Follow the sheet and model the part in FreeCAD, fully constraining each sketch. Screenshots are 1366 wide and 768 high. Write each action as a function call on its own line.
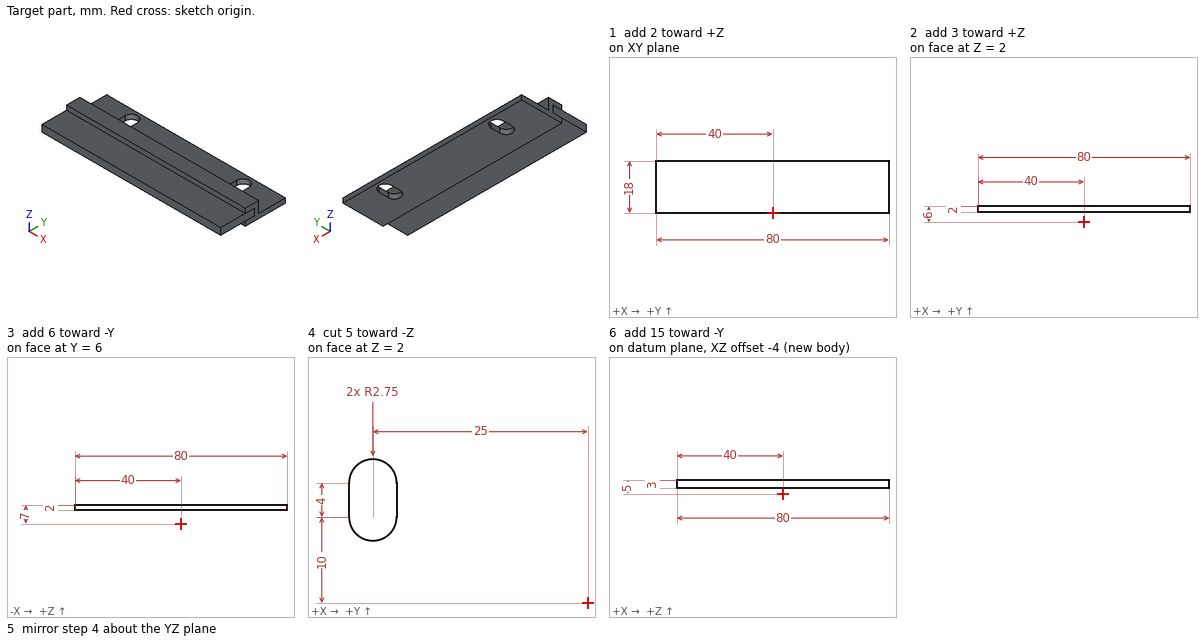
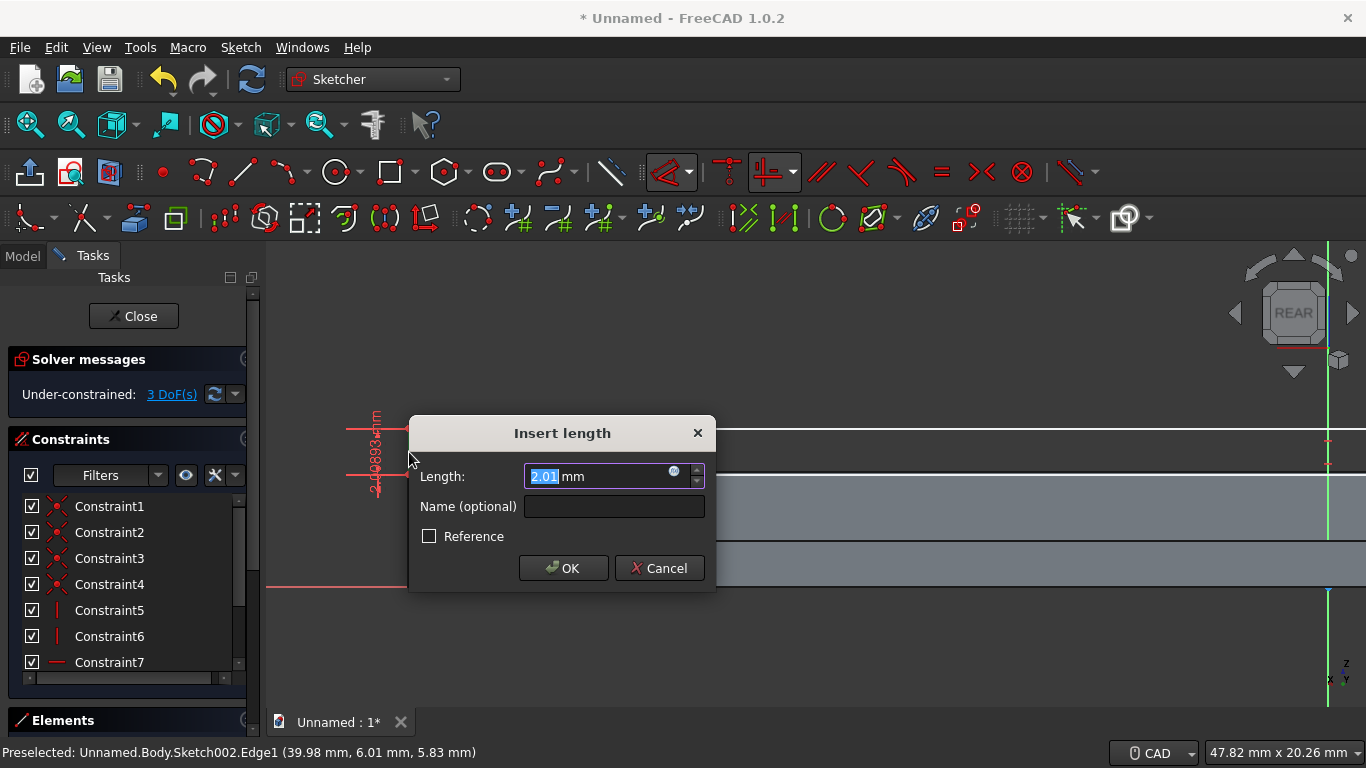
text(2)
key(Return)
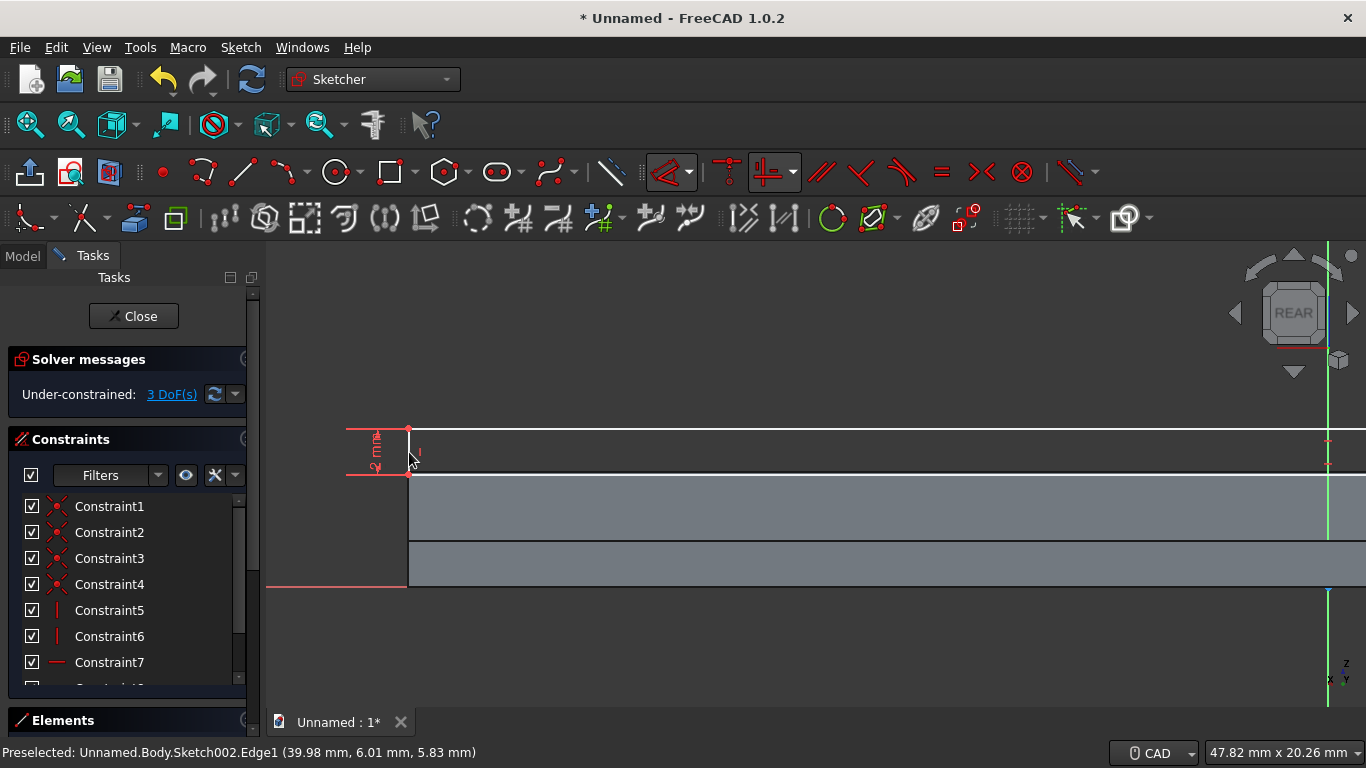
click(961, 475)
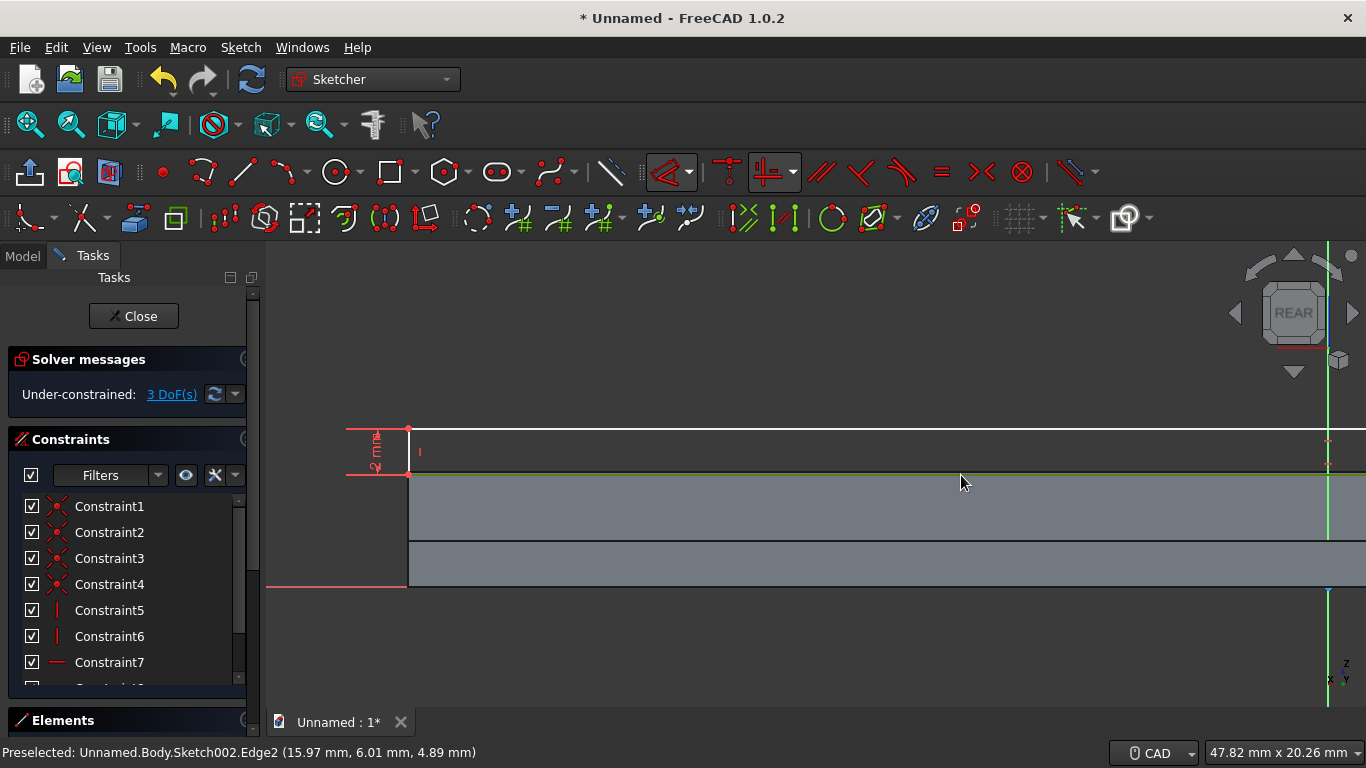
key(l)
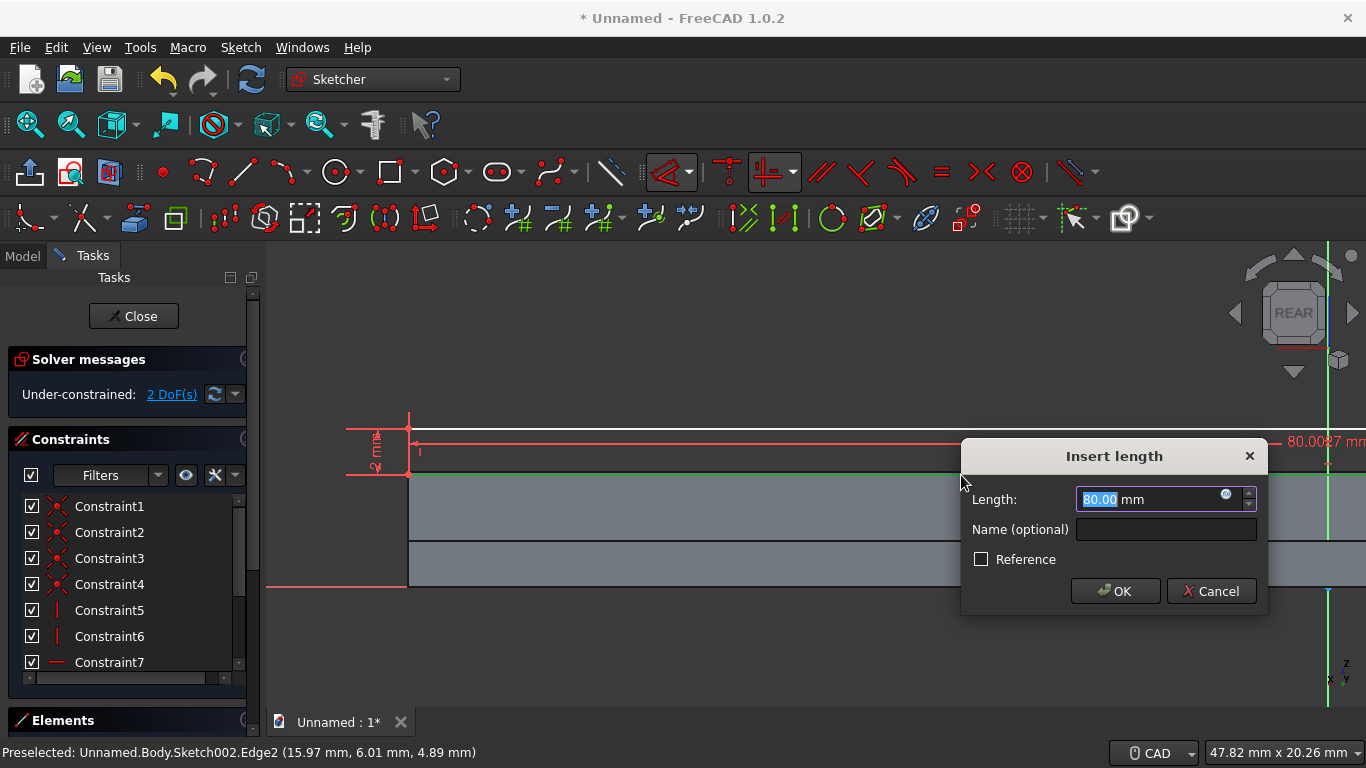
text(80)
key(Return)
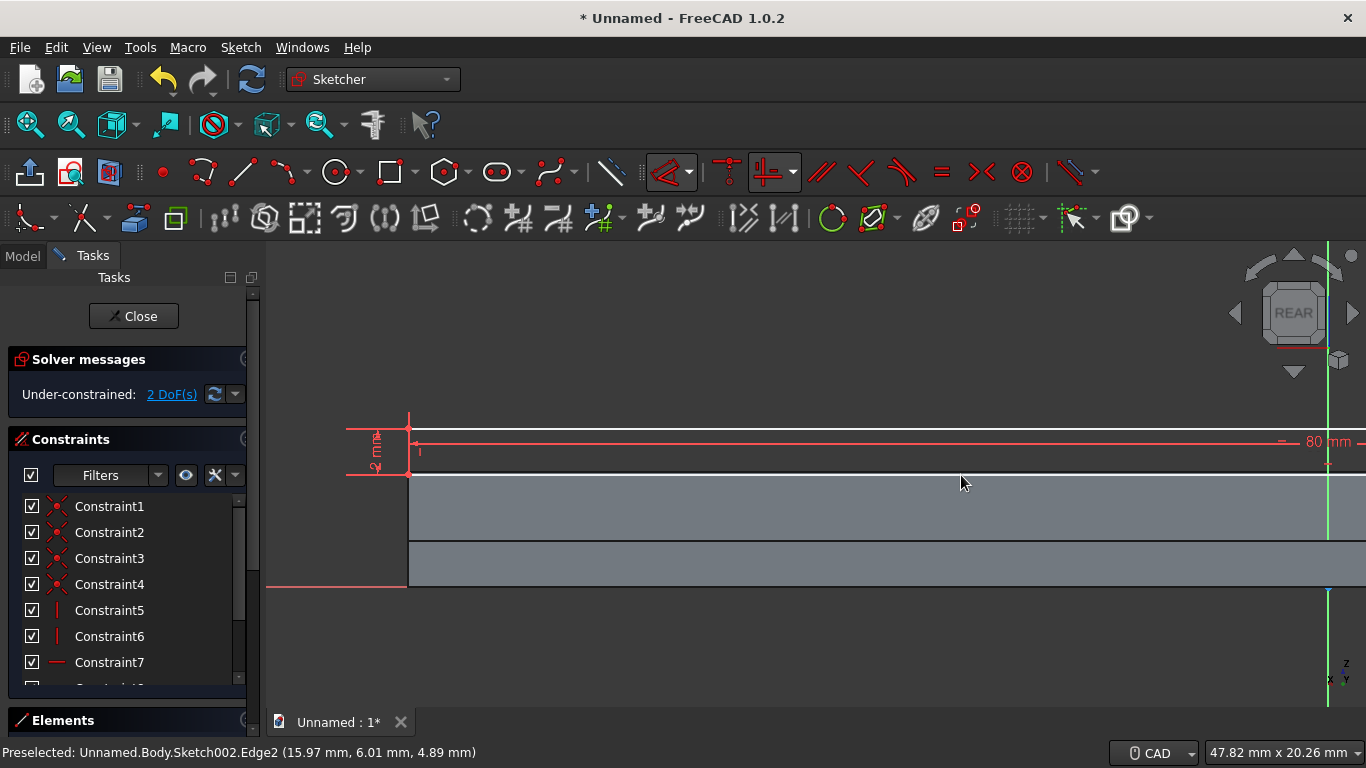
click(409, 429)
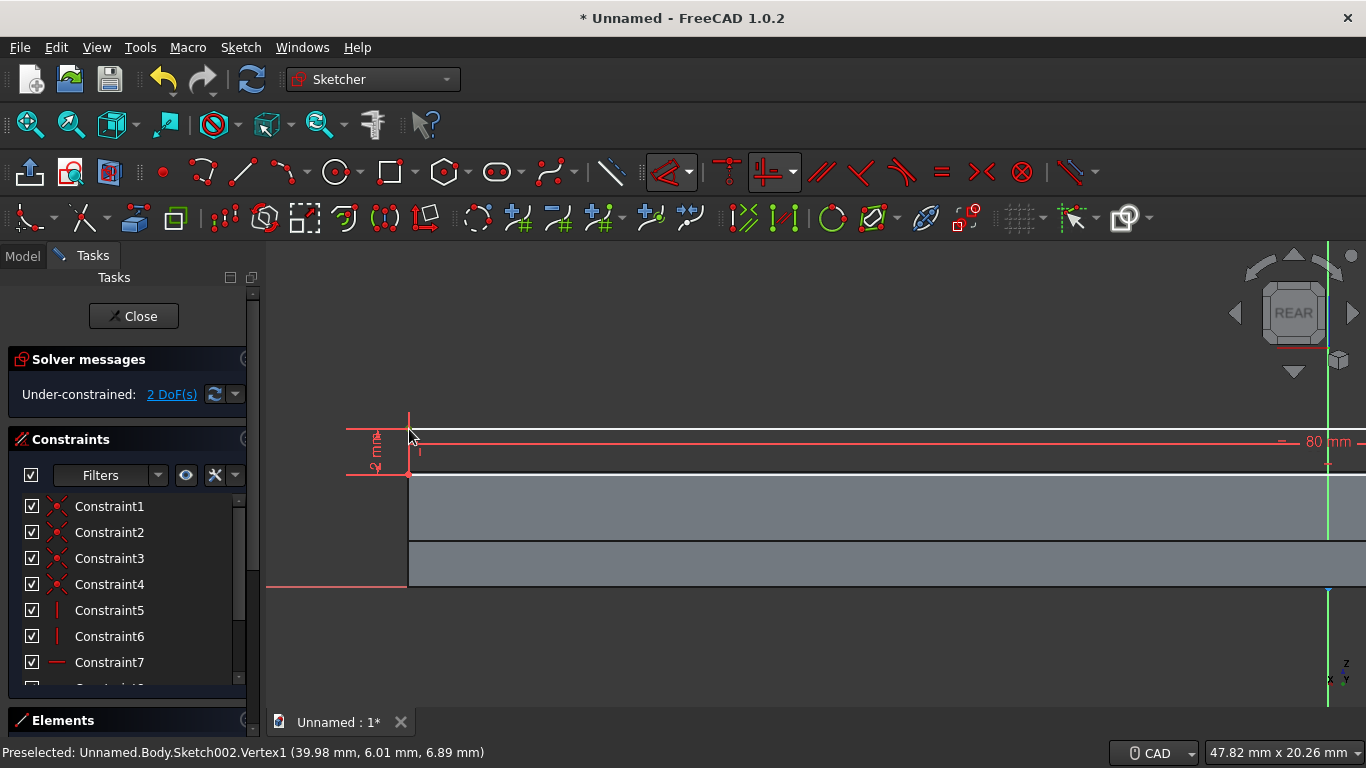
click(692, 172)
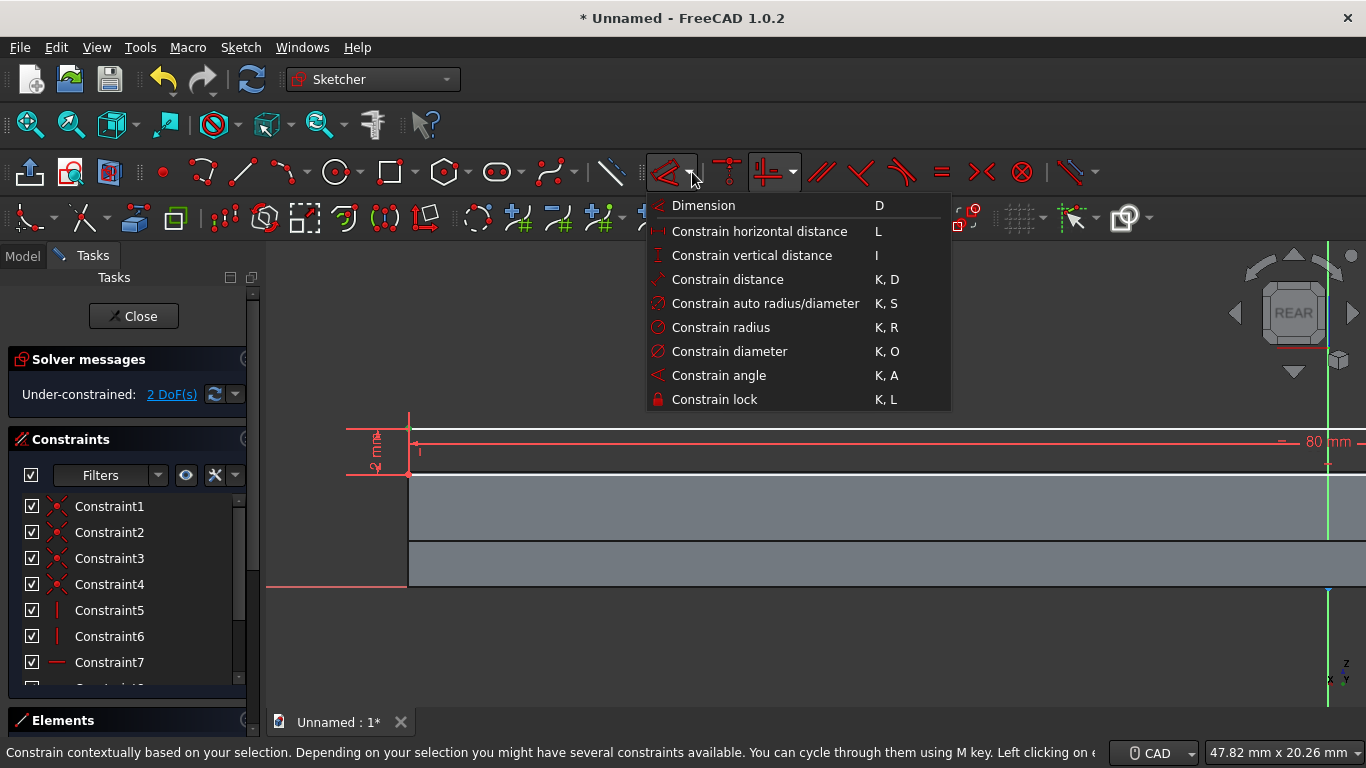
click(799, 255)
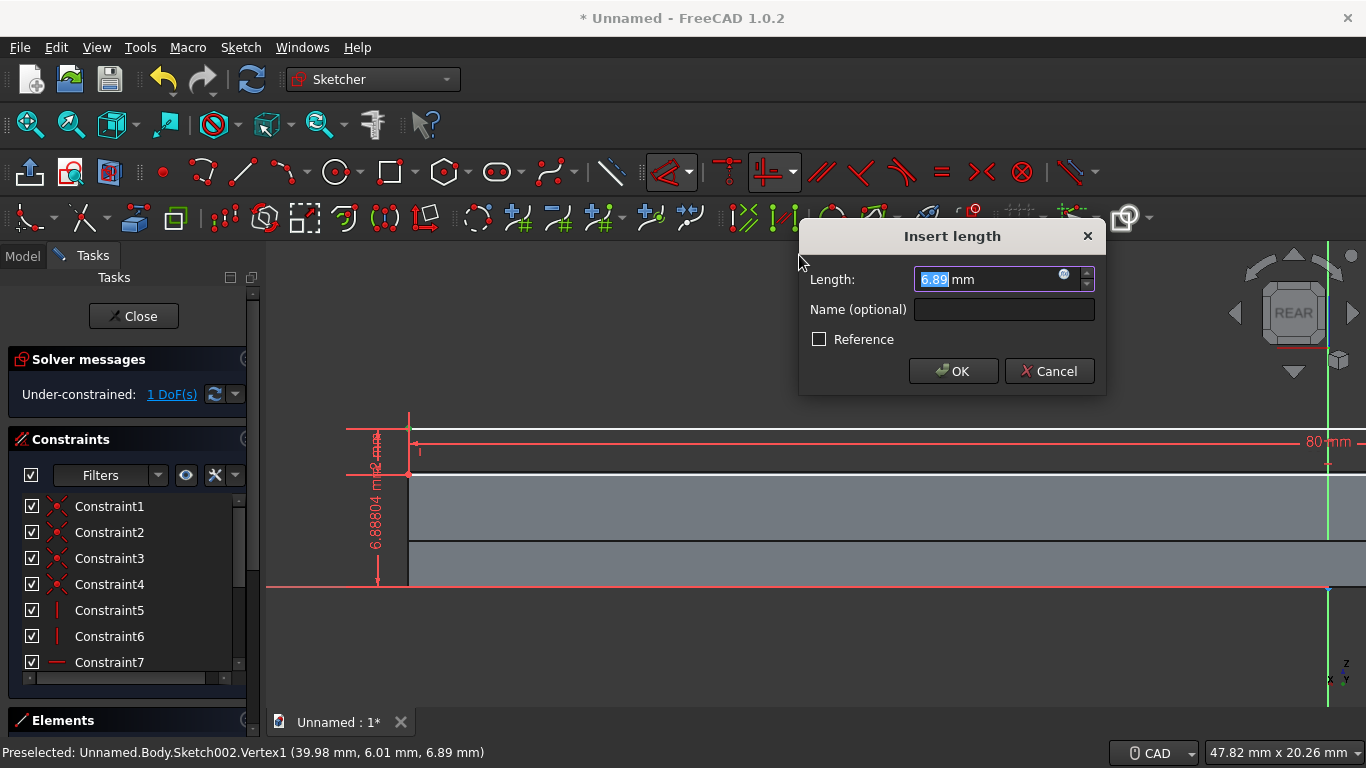
text(7)
key(Return)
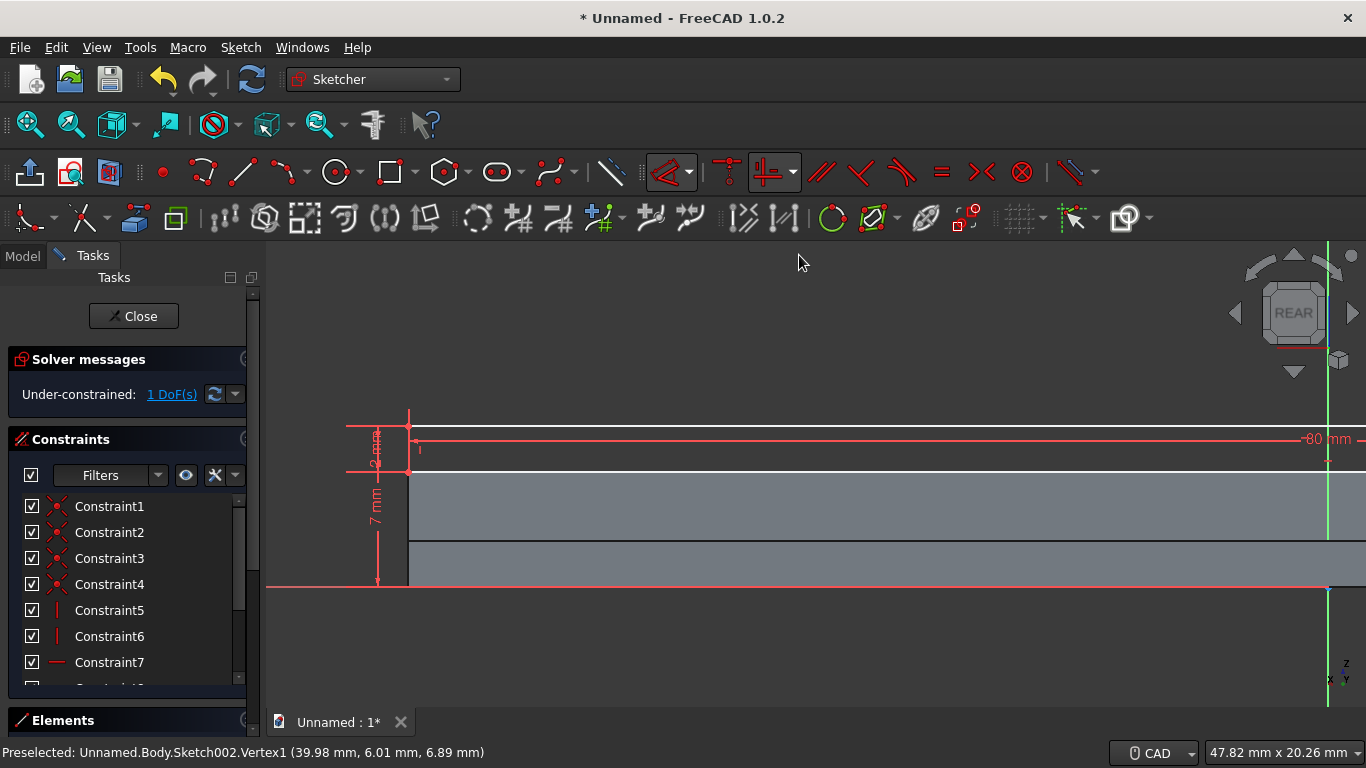
click(409, 426)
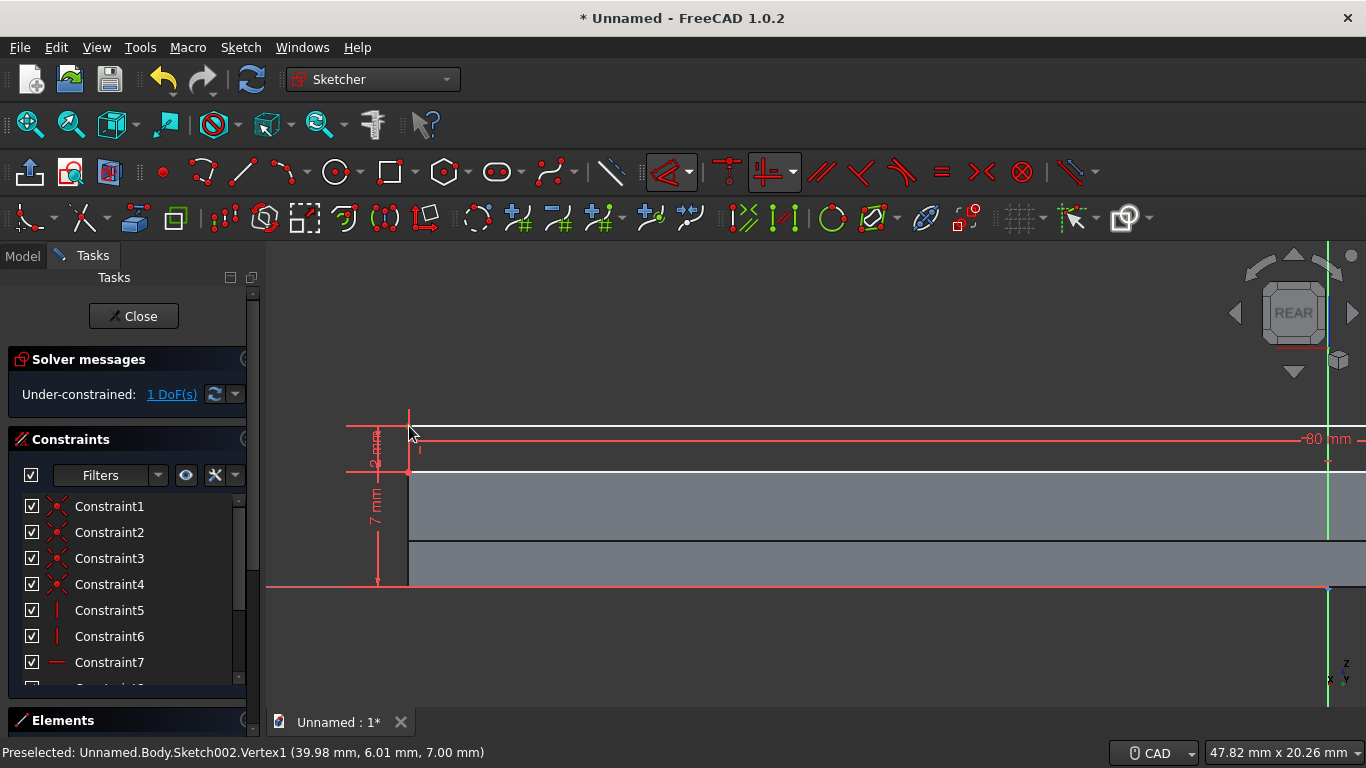
key(l)